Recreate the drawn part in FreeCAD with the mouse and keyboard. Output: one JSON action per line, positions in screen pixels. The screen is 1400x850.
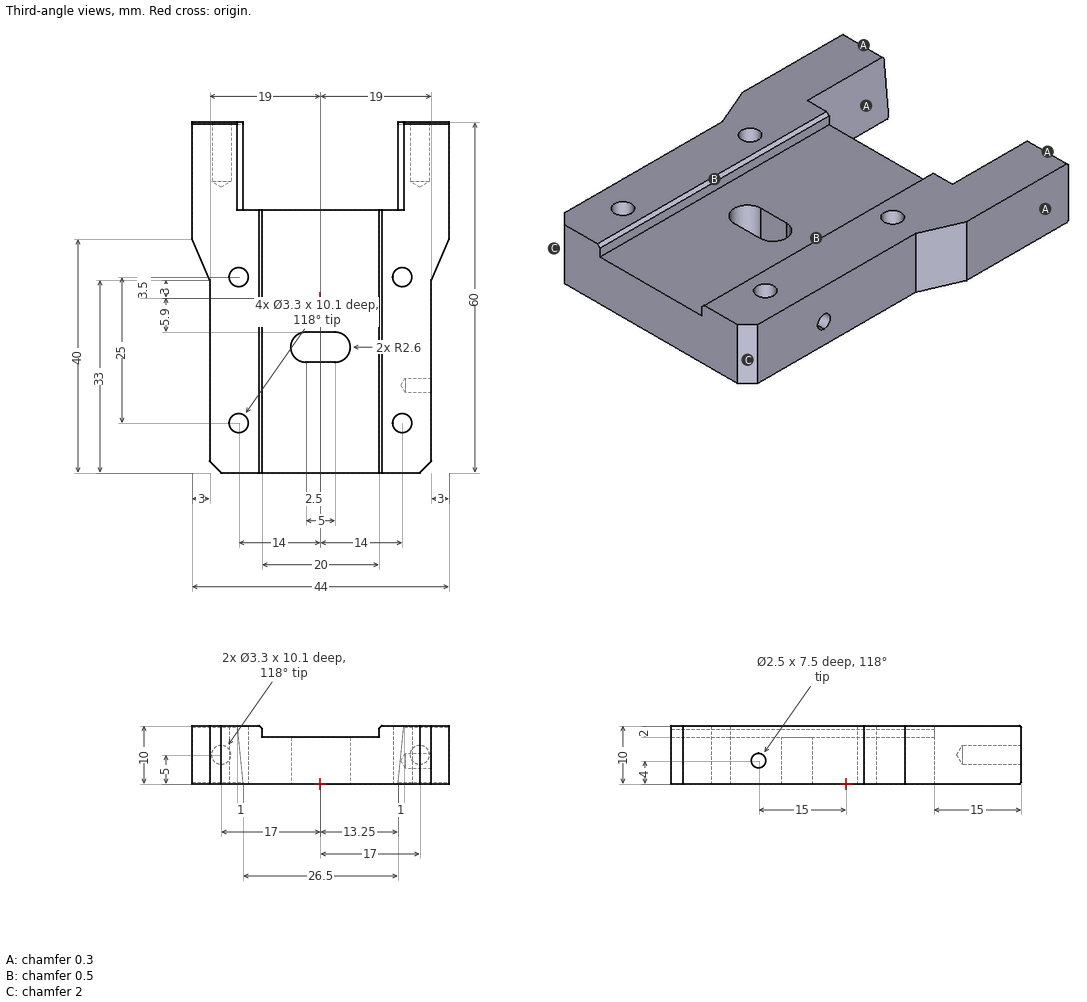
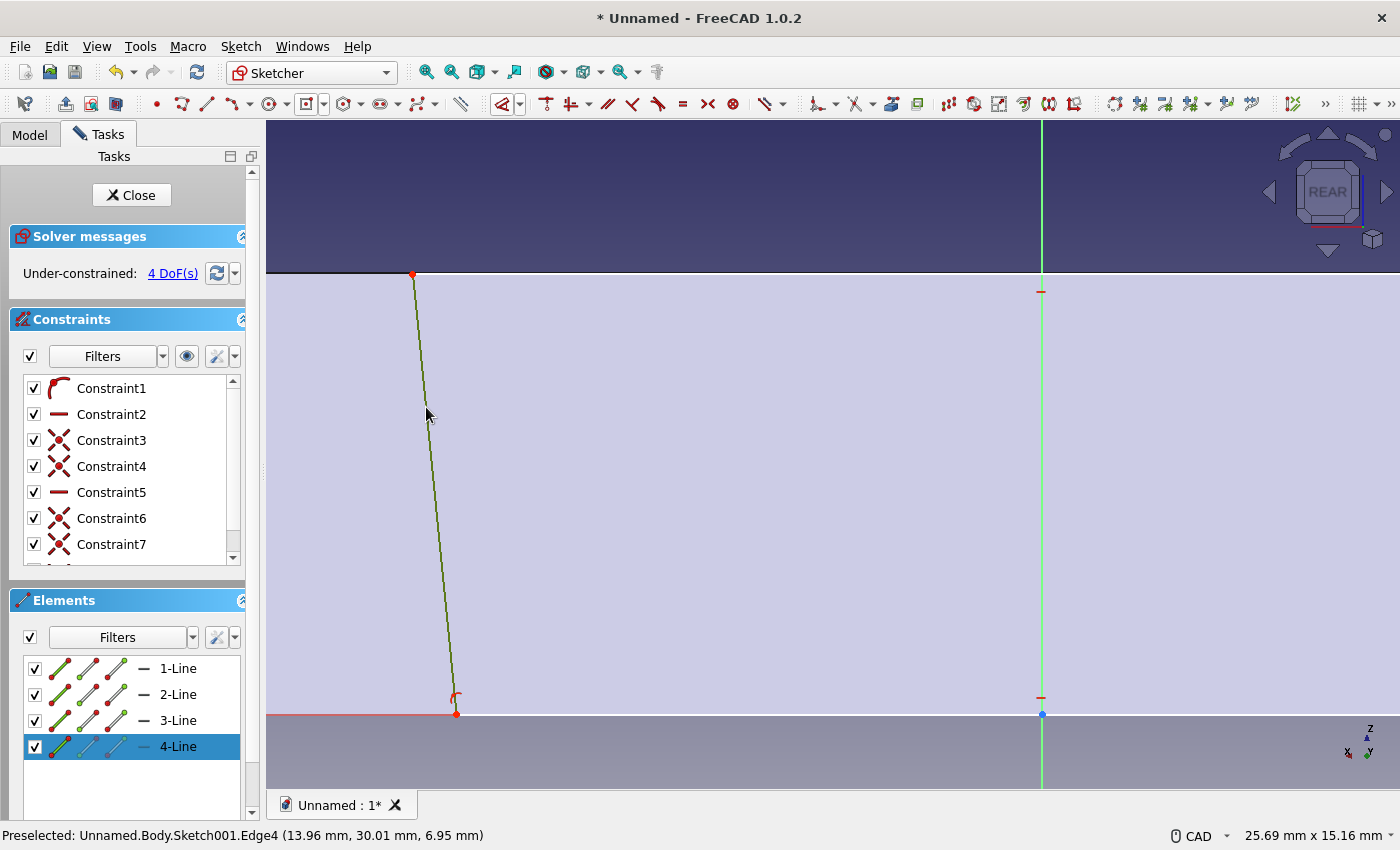
{"action": "left_click", "coordinate": [520, 104]}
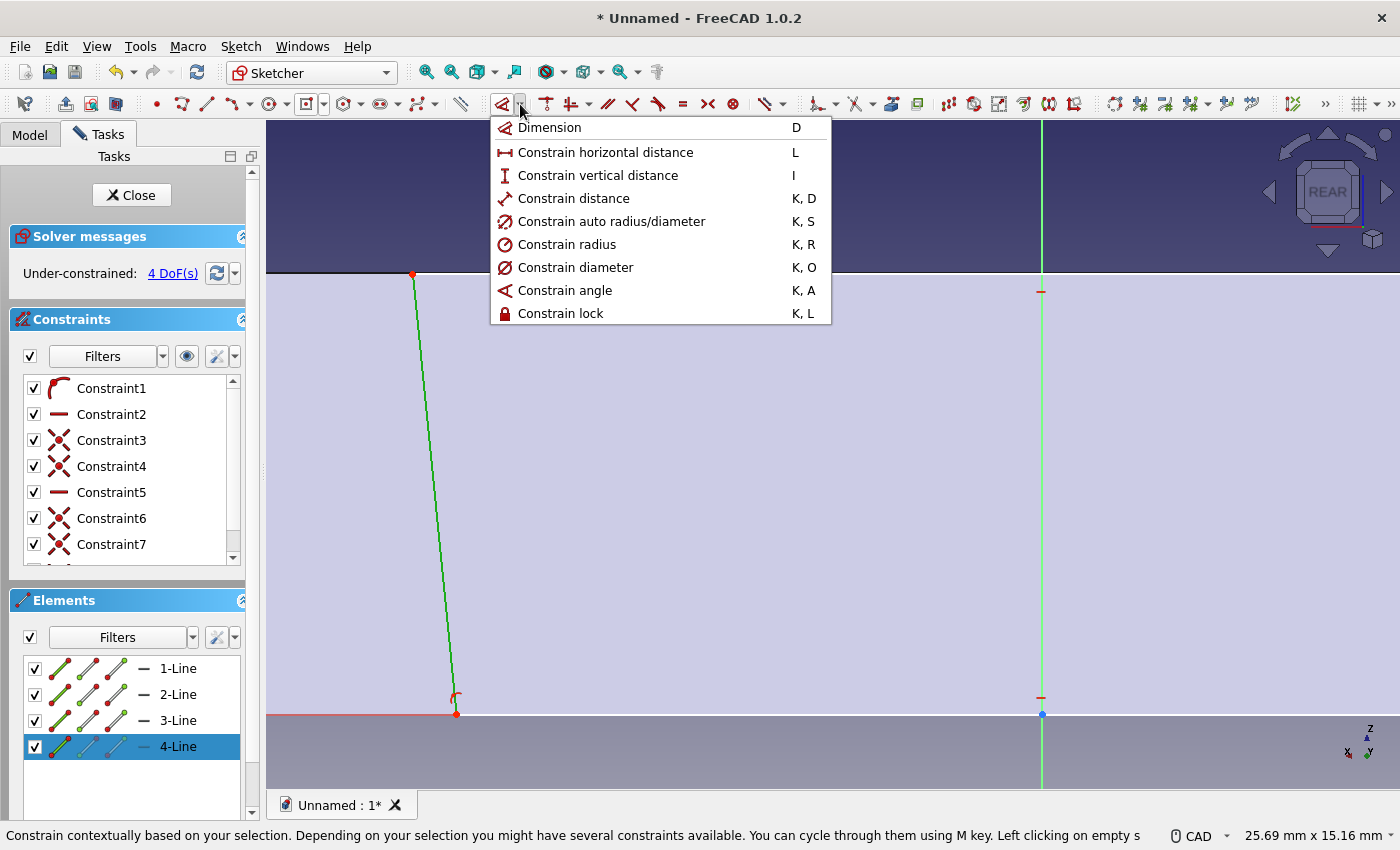
{"action": "left_click", "coordinate": [661, 152]}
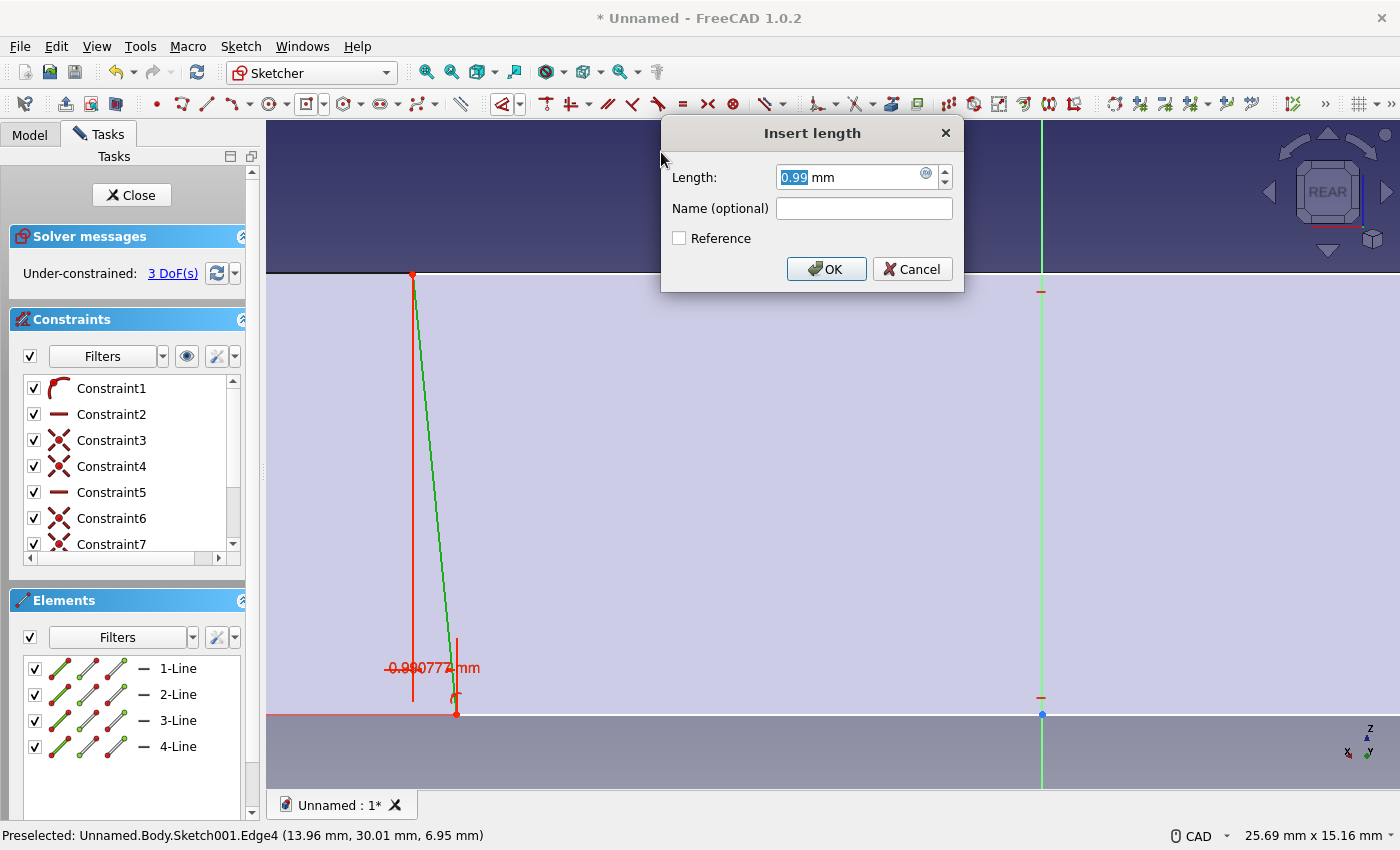
{"action": "type", "text": "1"}
{"action": "key", "text": "Return"}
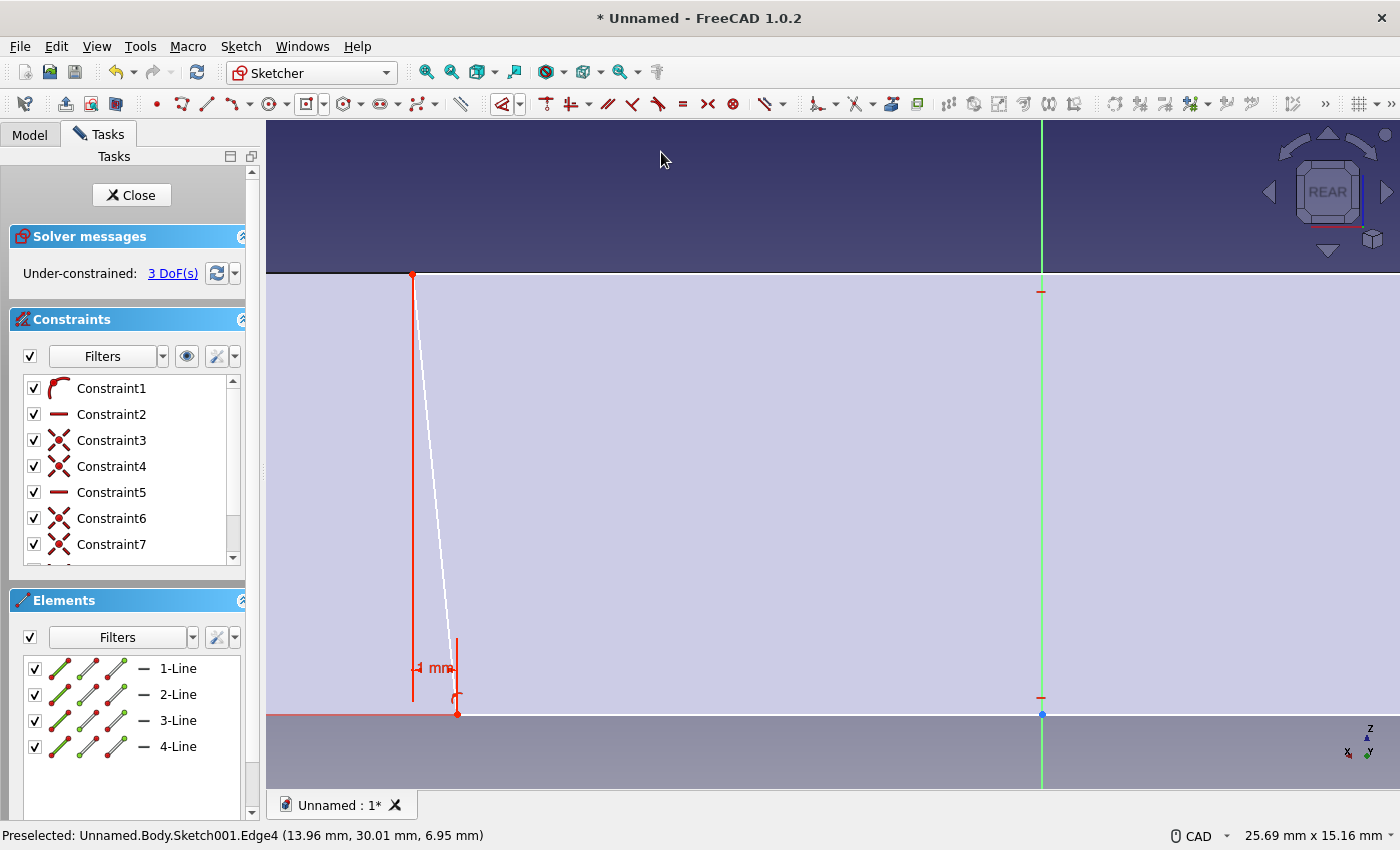
{"action": "scroll", "coordinate": [427, 406], "scroll_direction": "down", "scroll_amount": 3}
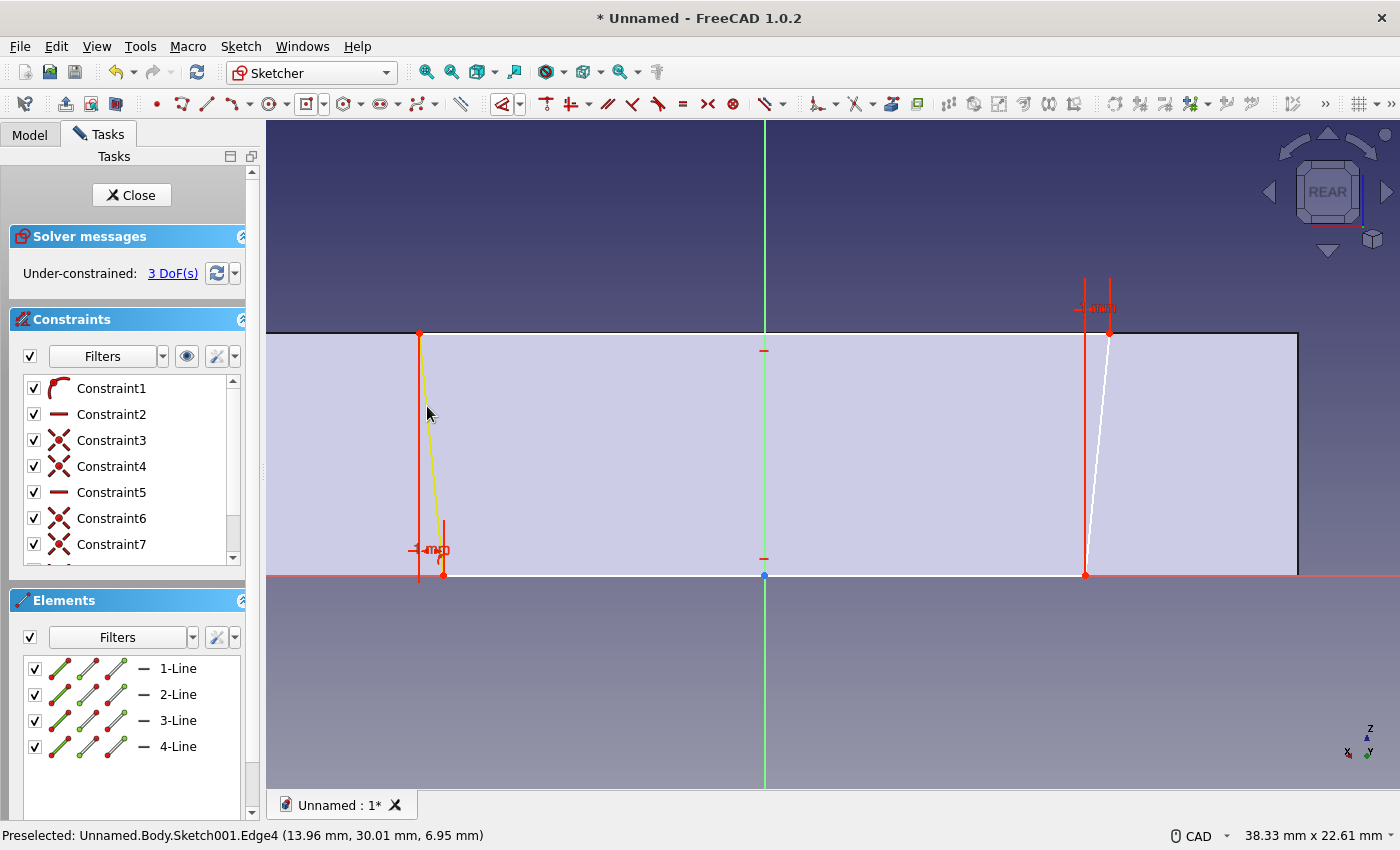
{"action": "left_click", "coordinate": [1110, 334]}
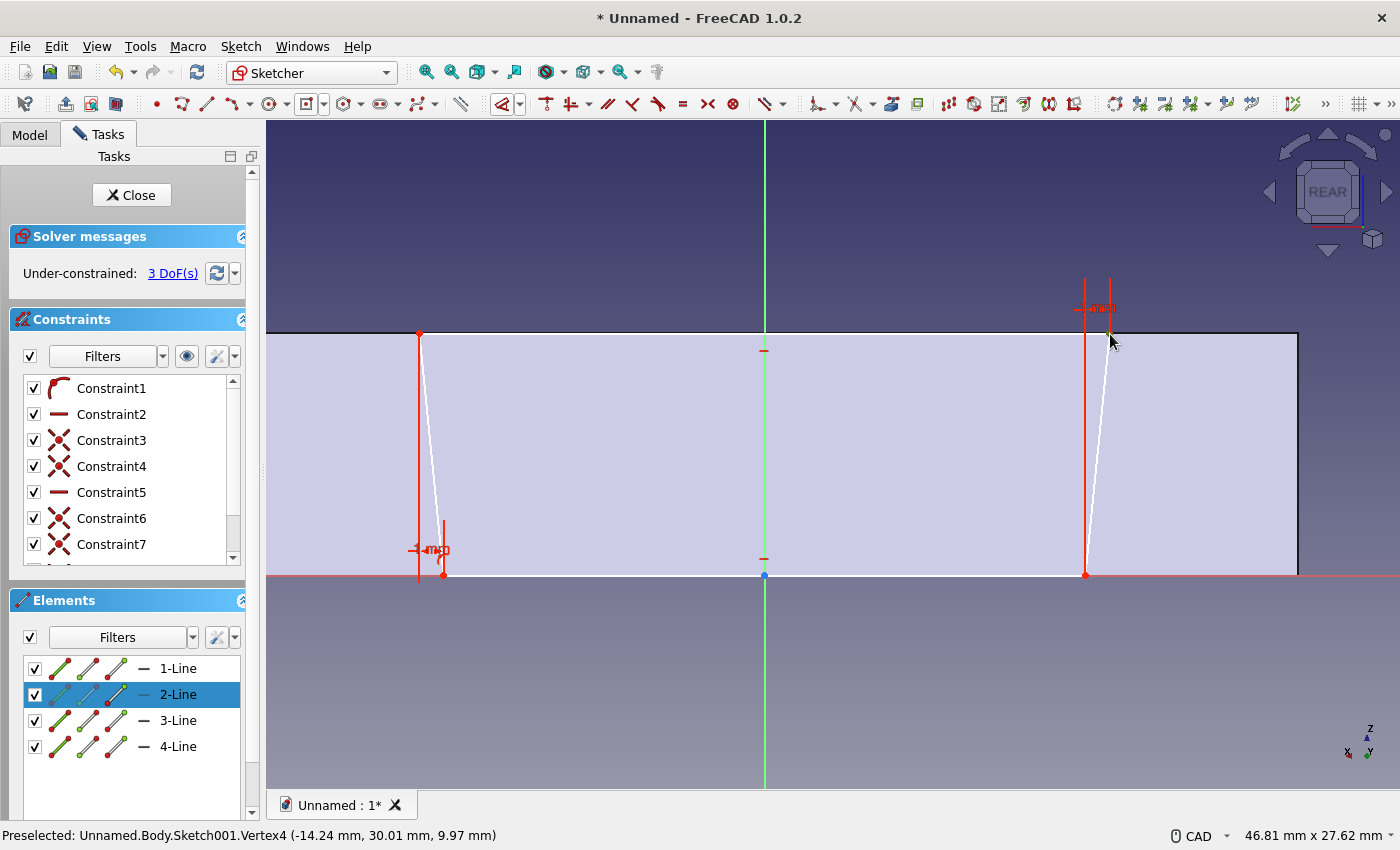
{"action": "key", "text": "i"}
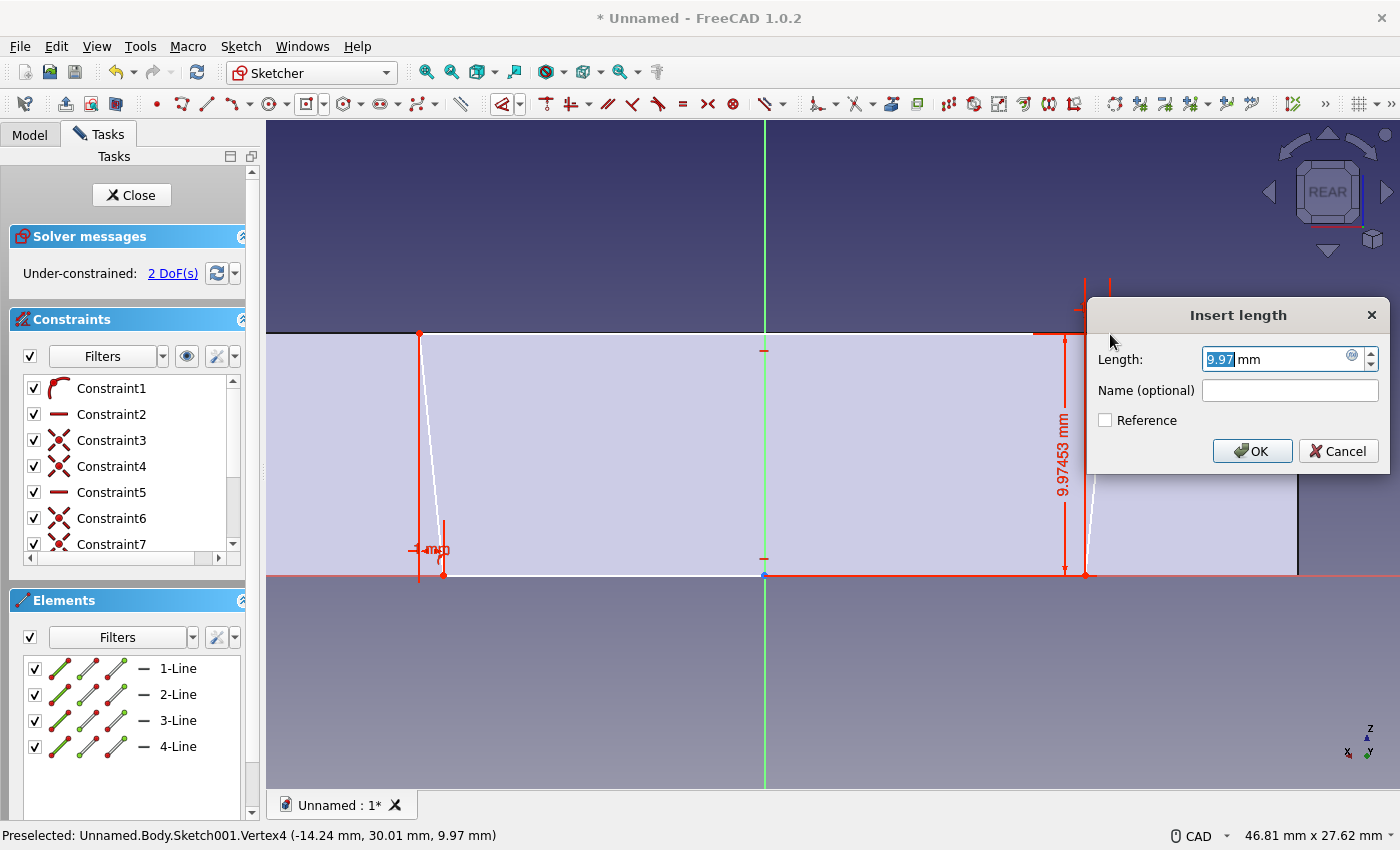
{"action": "type", "text": "10"}
{"action": "key", "text": "Return"}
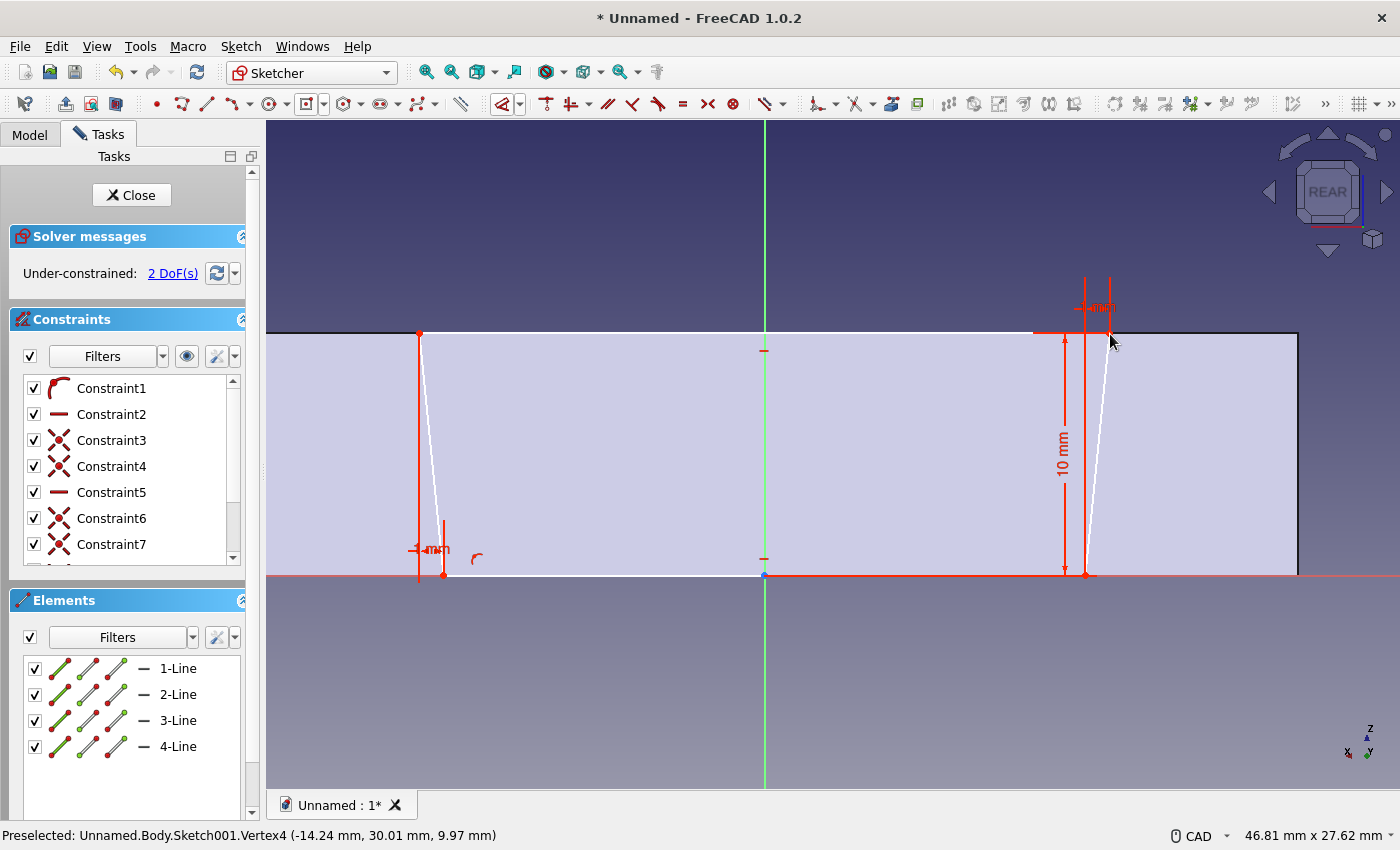
{"action": "left_click", "coordinate": [636, 576]}